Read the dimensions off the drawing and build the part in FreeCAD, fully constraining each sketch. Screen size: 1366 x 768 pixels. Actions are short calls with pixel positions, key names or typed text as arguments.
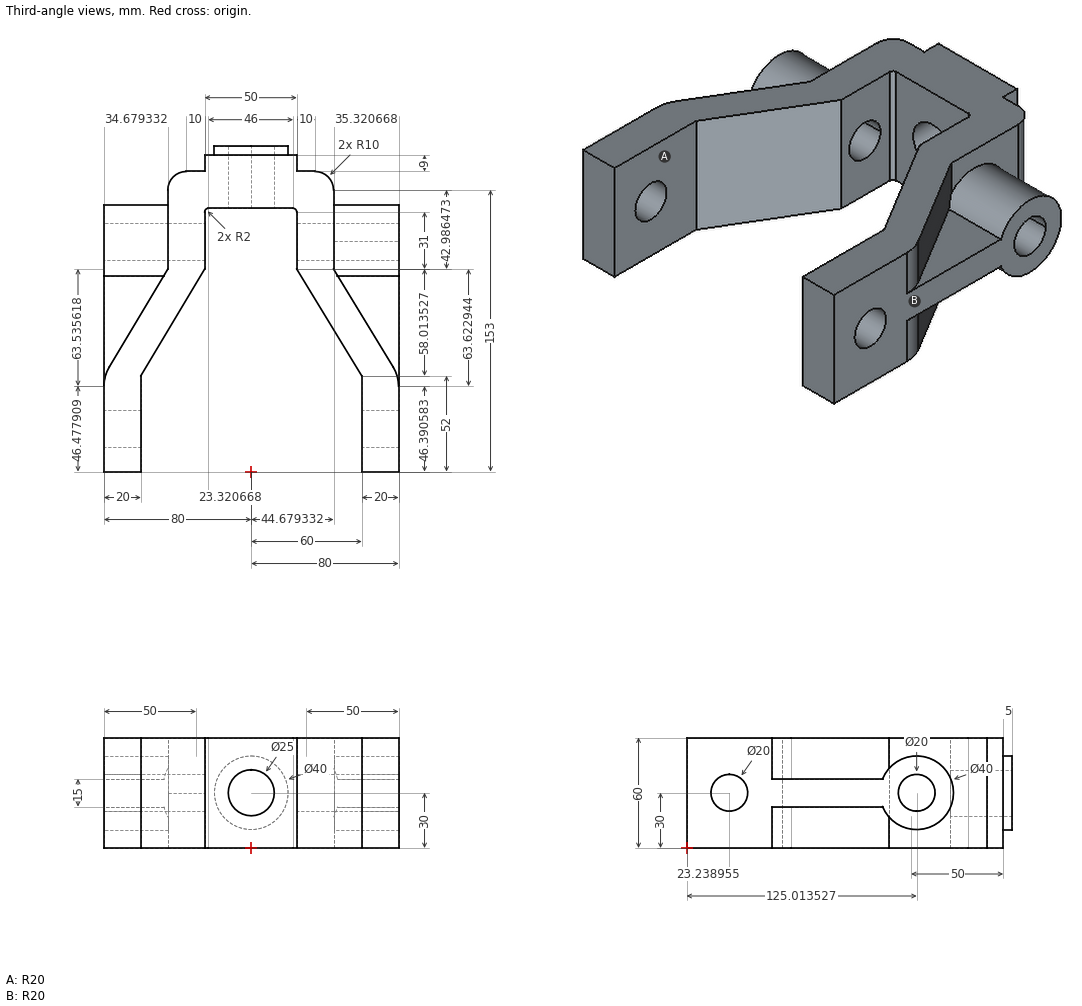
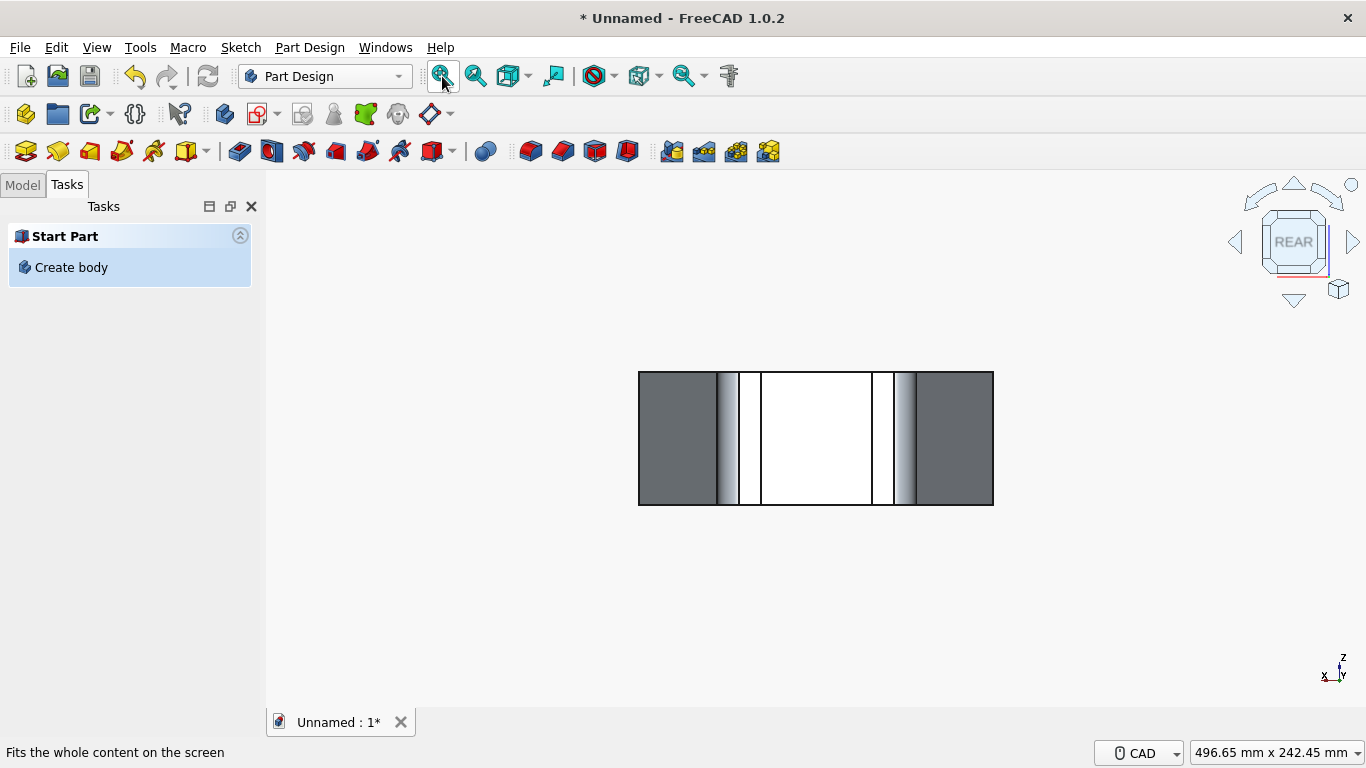
click(817, 438)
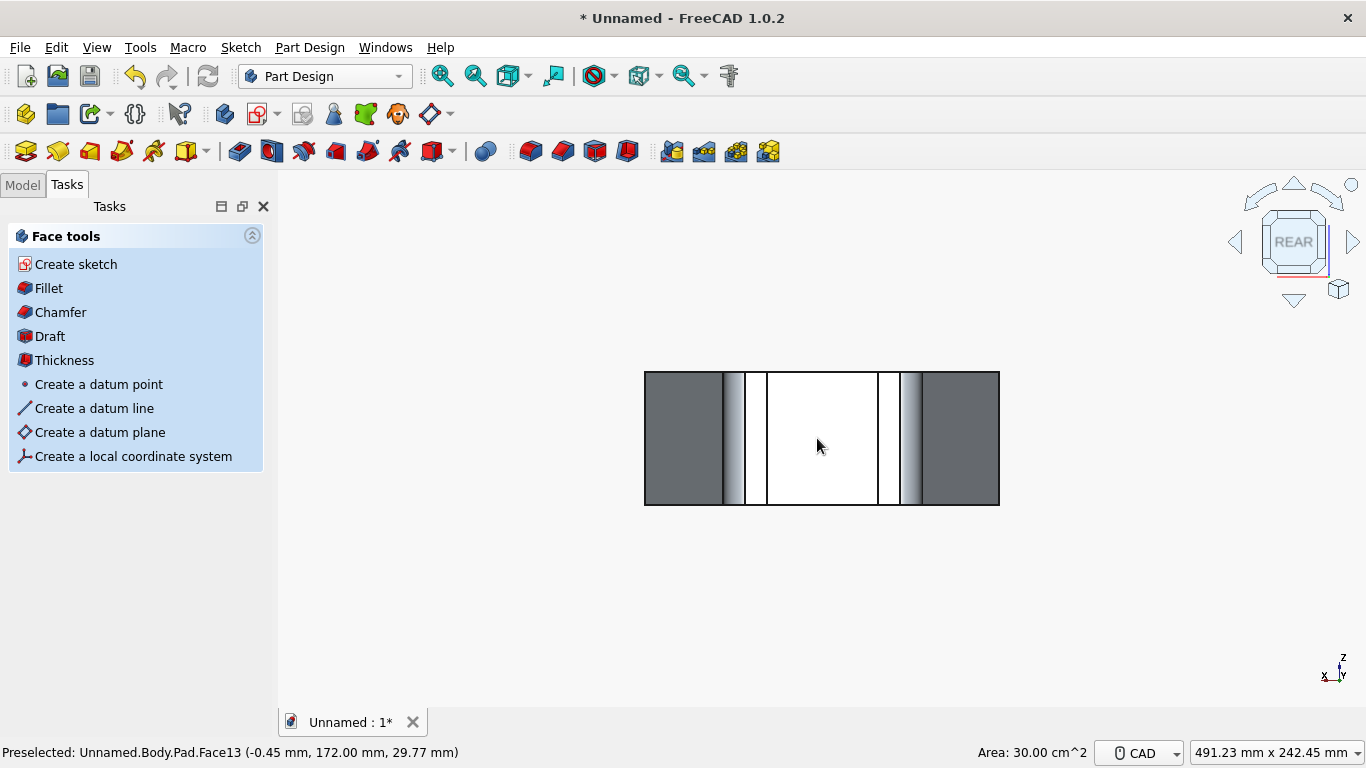
click(258, 114)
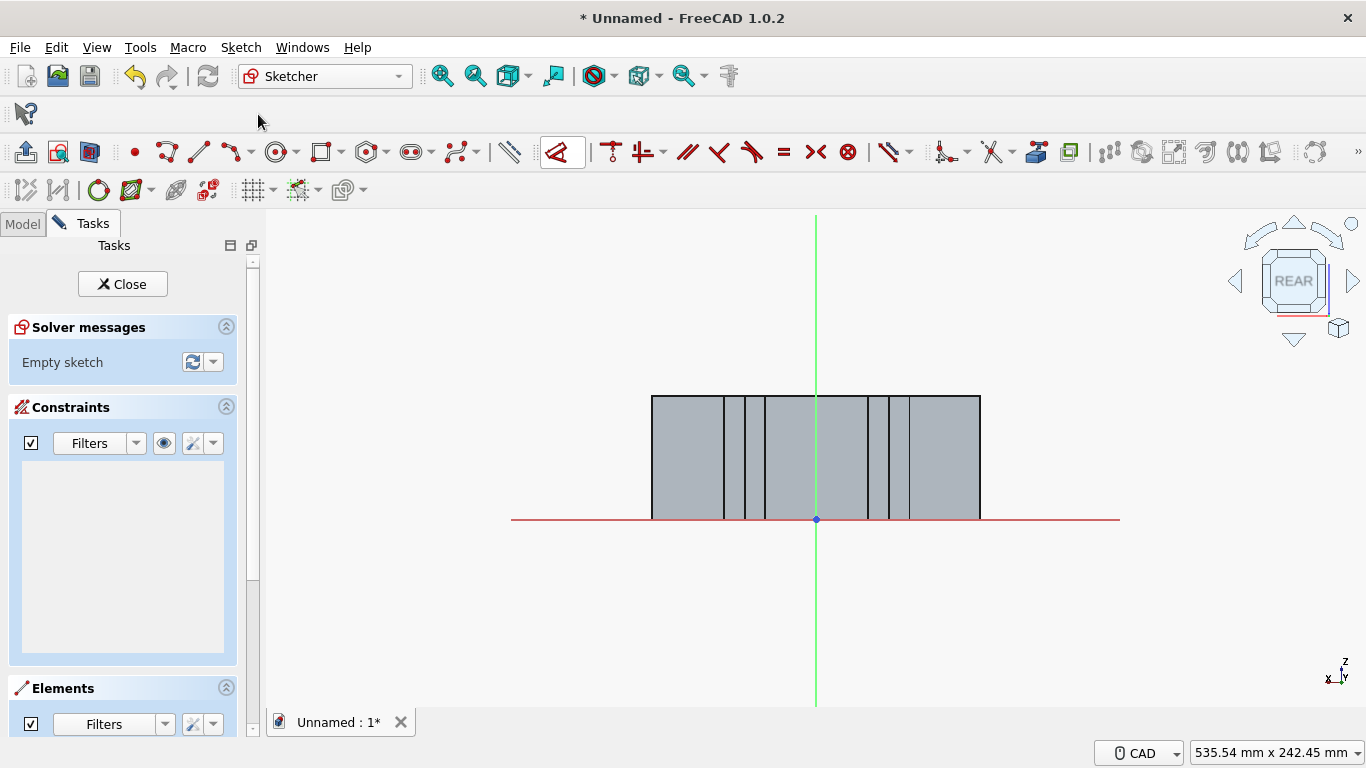
scroll(846, 473, up, 6)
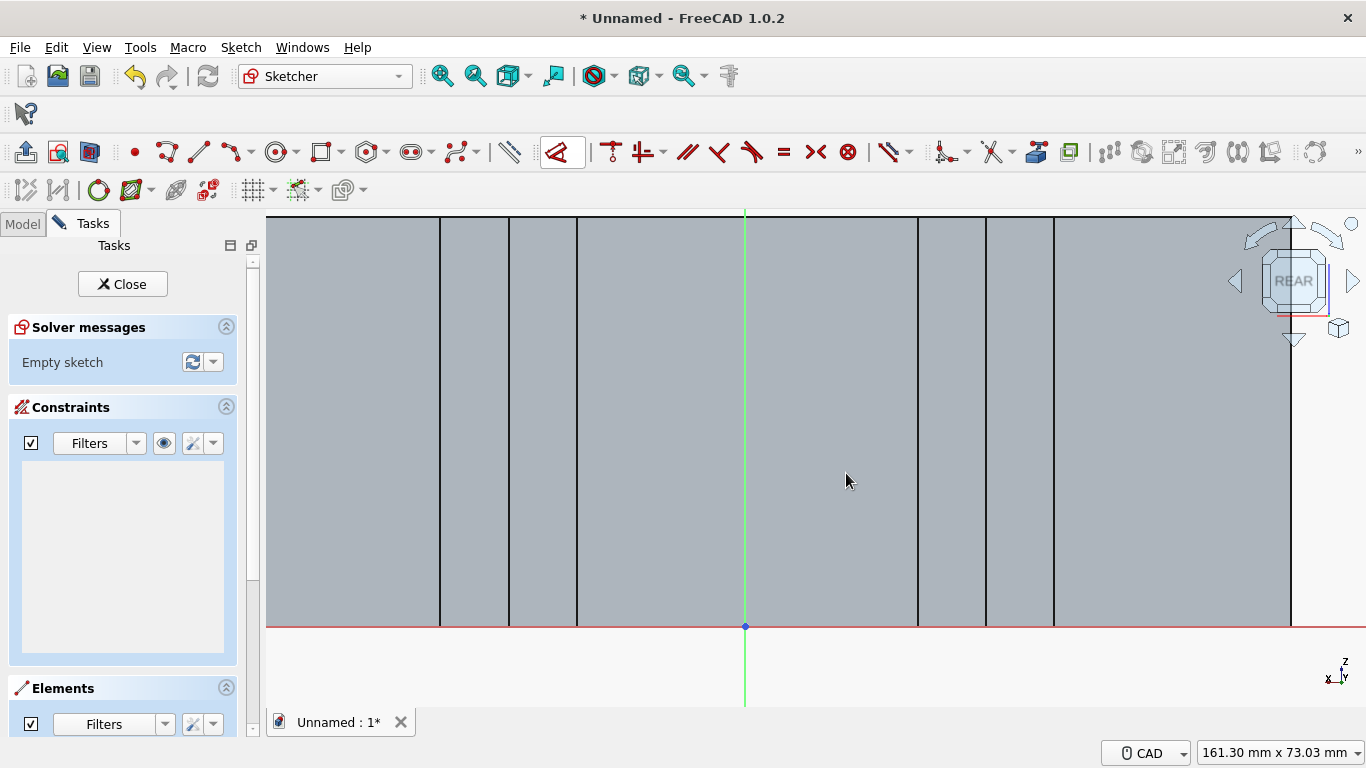
click(276, 152)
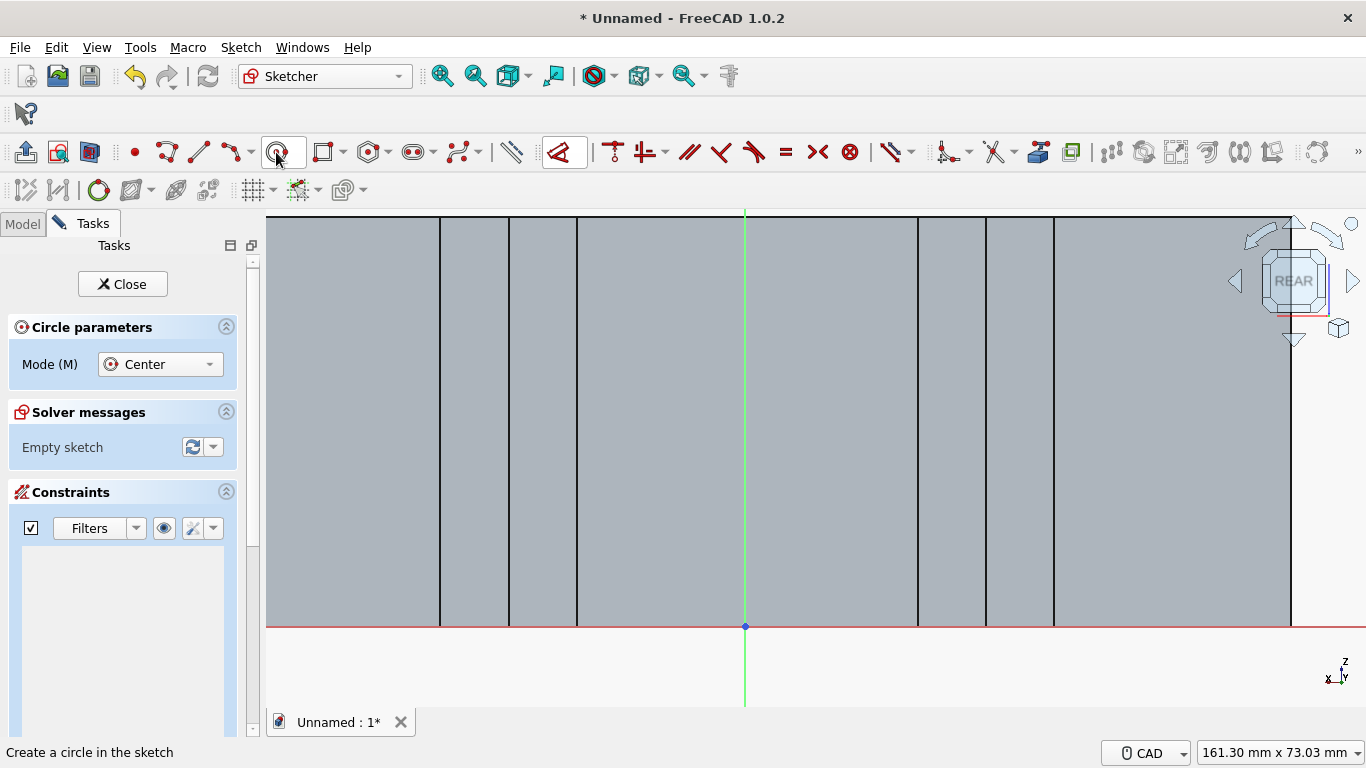
click(745, 422)
click(842, 326)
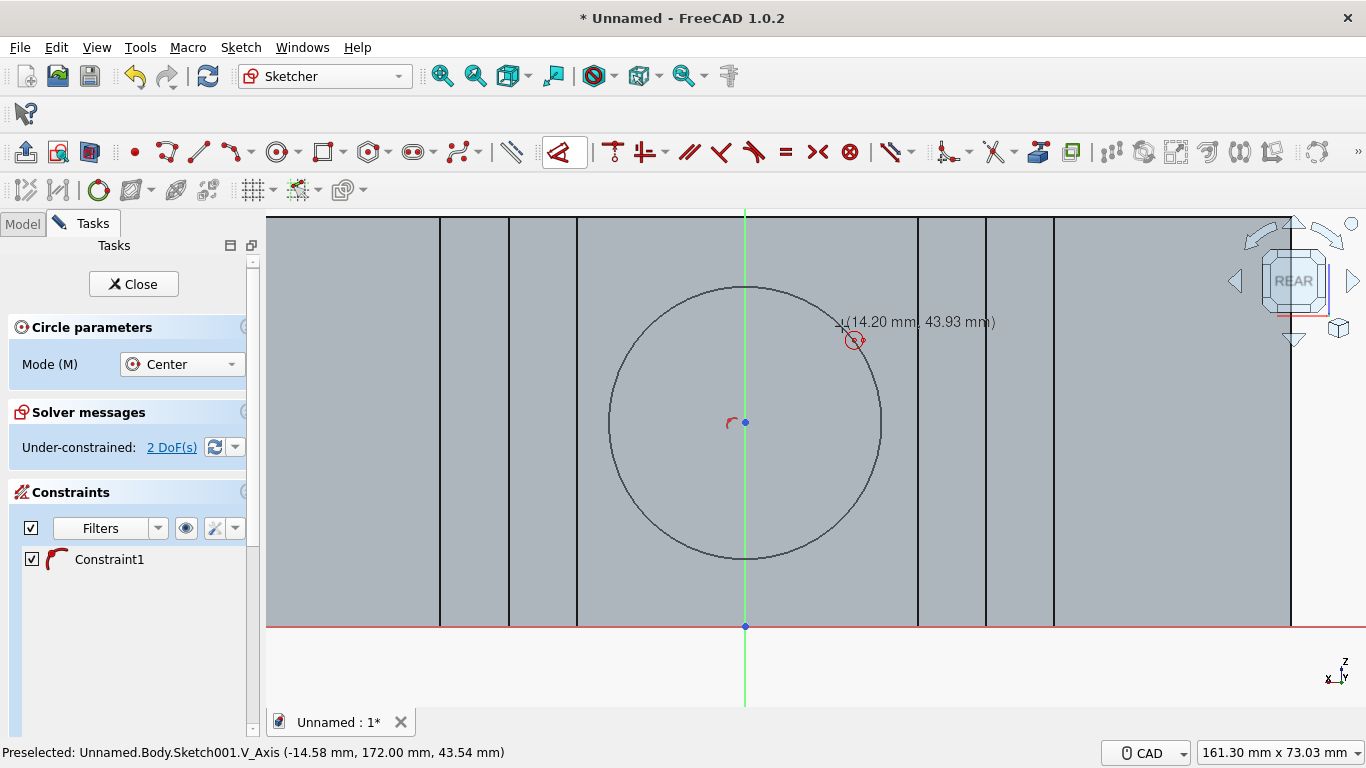
click(745, 423)
click(805, 362)
key(Escape)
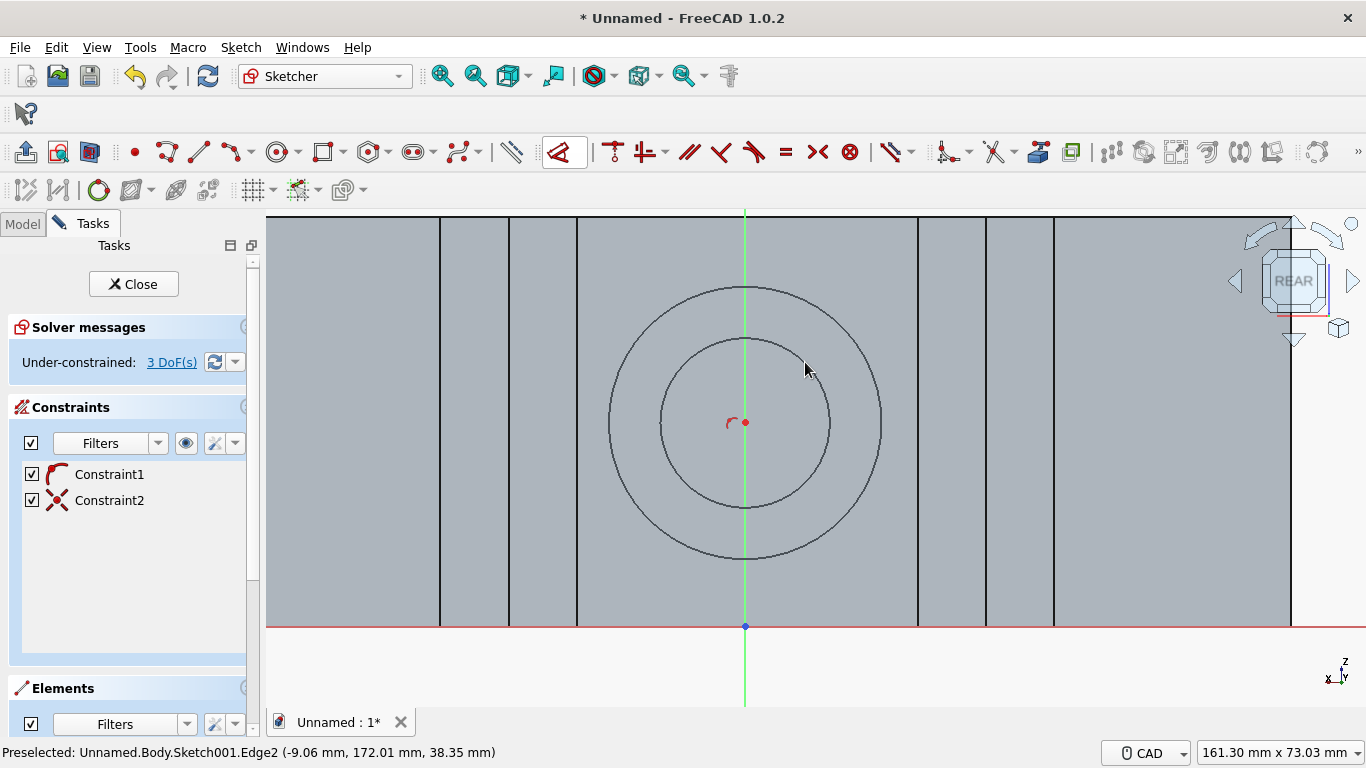
click(841, 326)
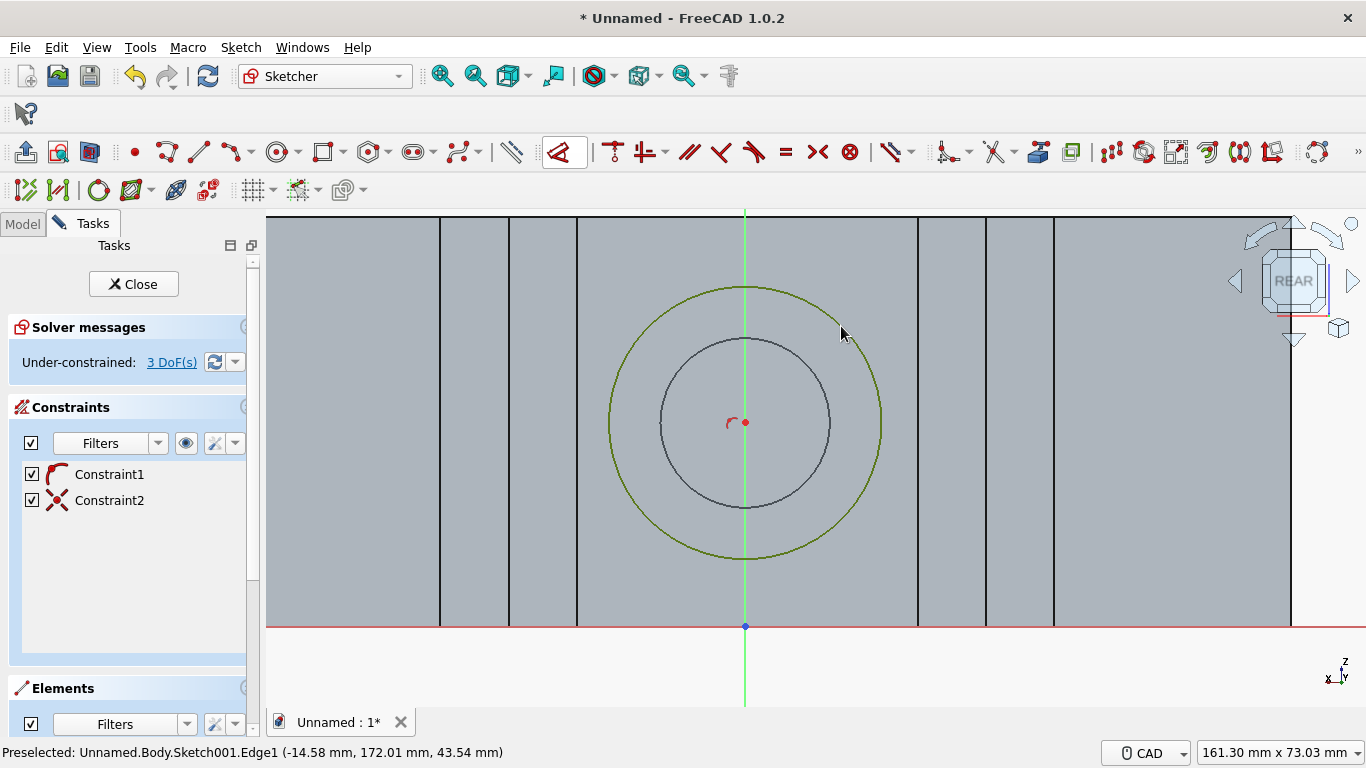
key(k)
key(o)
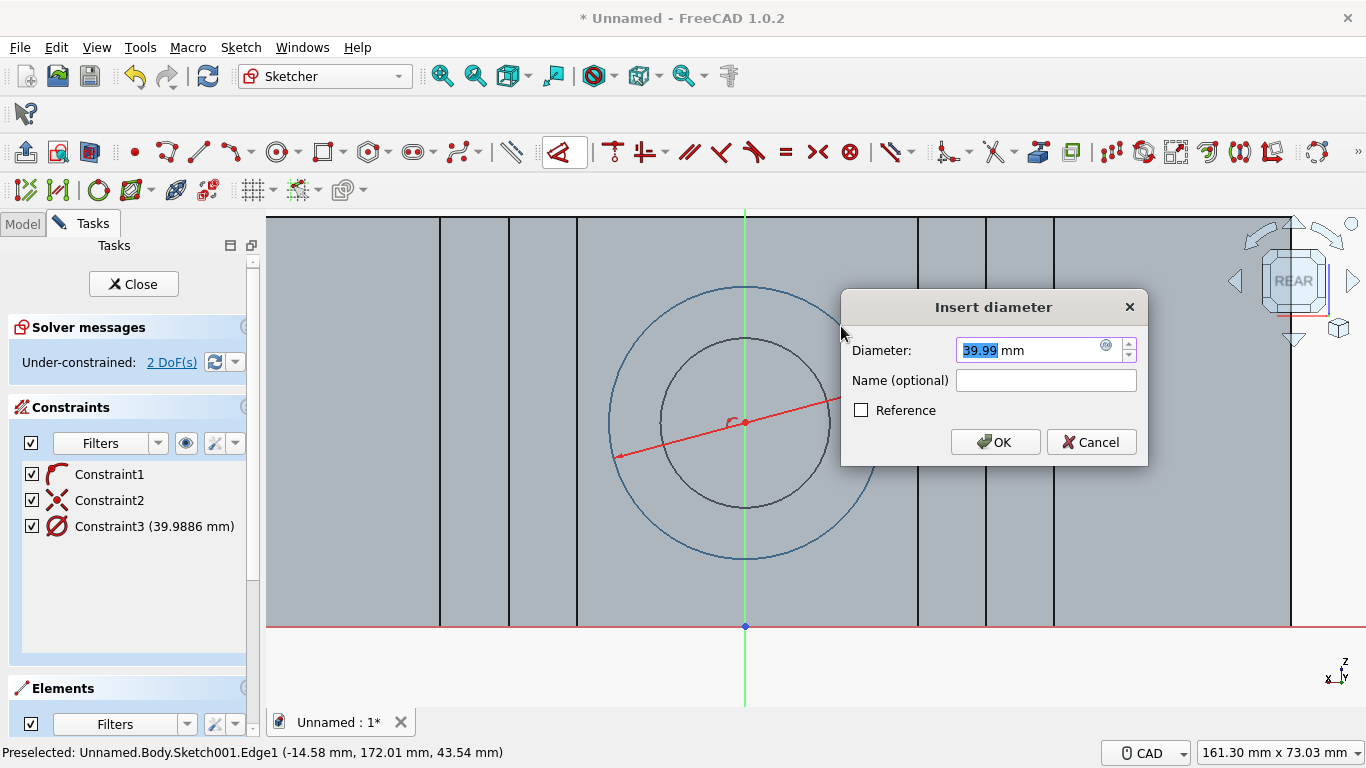
text(40)
key(Return)